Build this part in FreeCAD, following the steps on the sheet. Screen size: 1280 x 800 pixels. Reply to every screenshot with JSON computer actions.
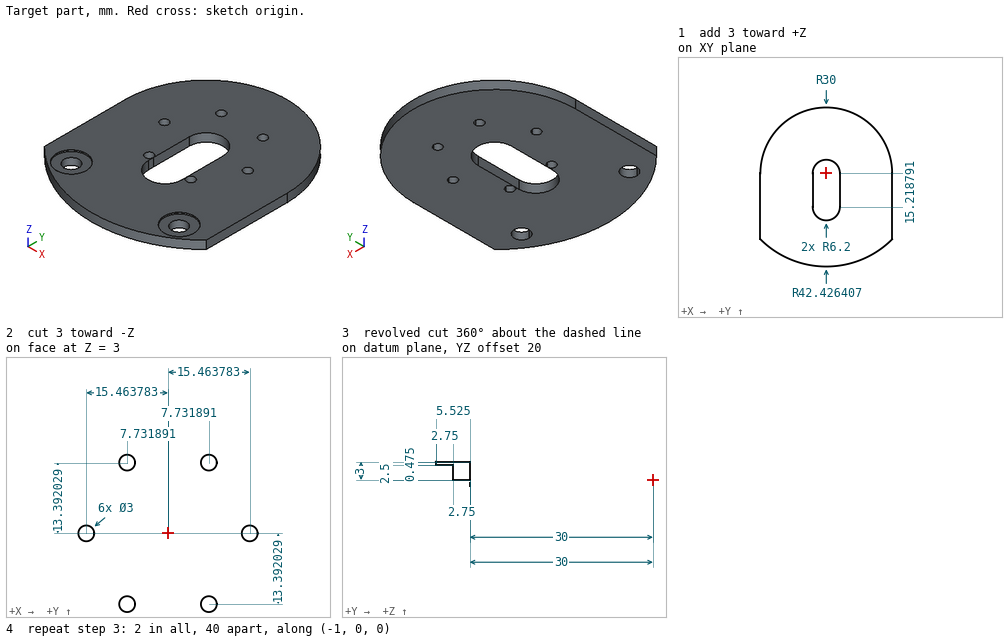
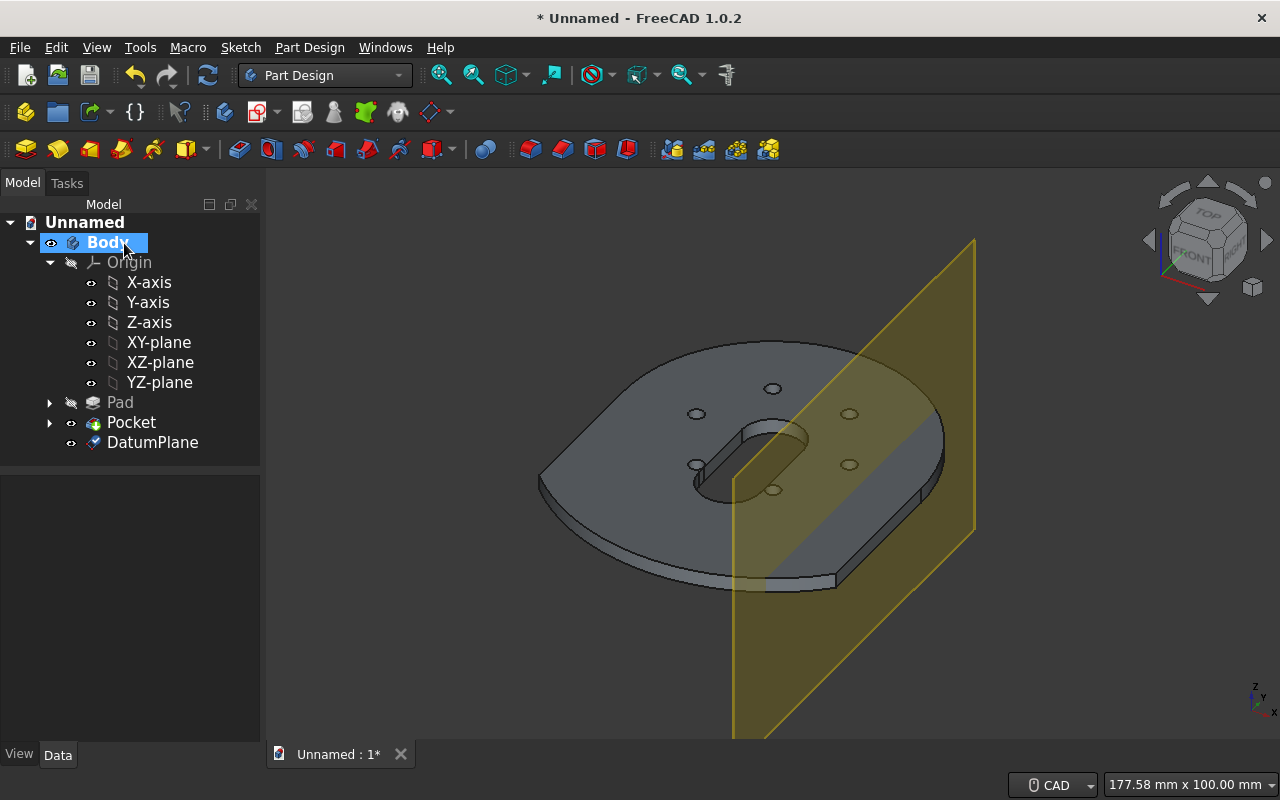
{"action": "left_click", "coordinate": [116, 443]}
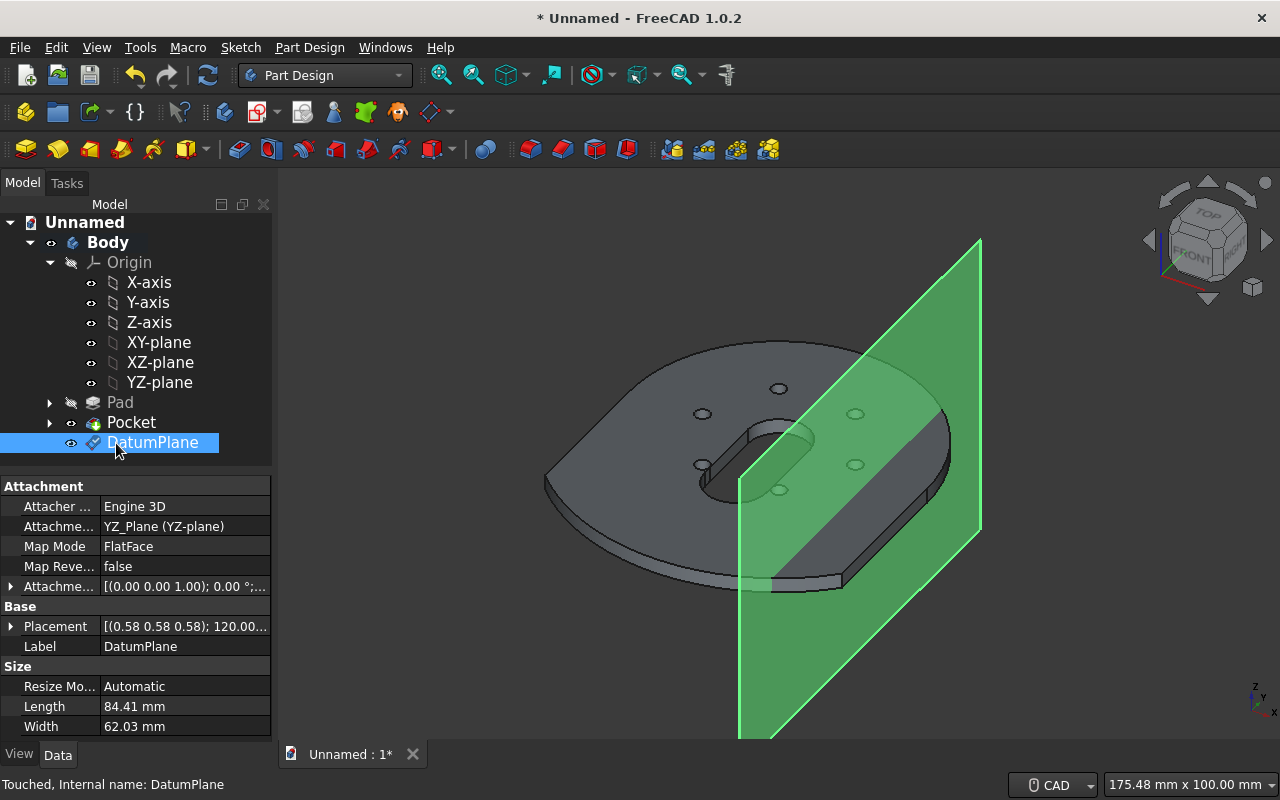
{"action": "left_click", "coordinate": [258, 112]}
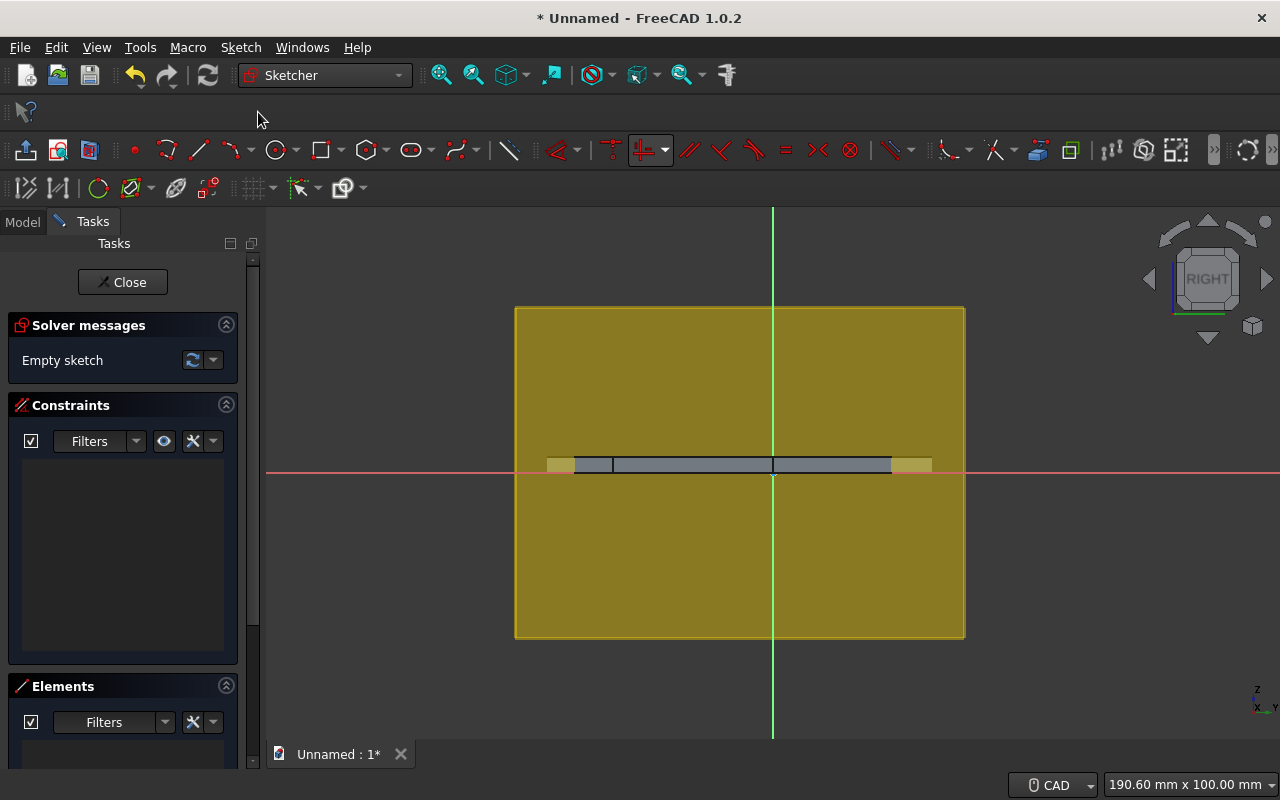
{"action": "left_click", "coordinate": [90, 150]}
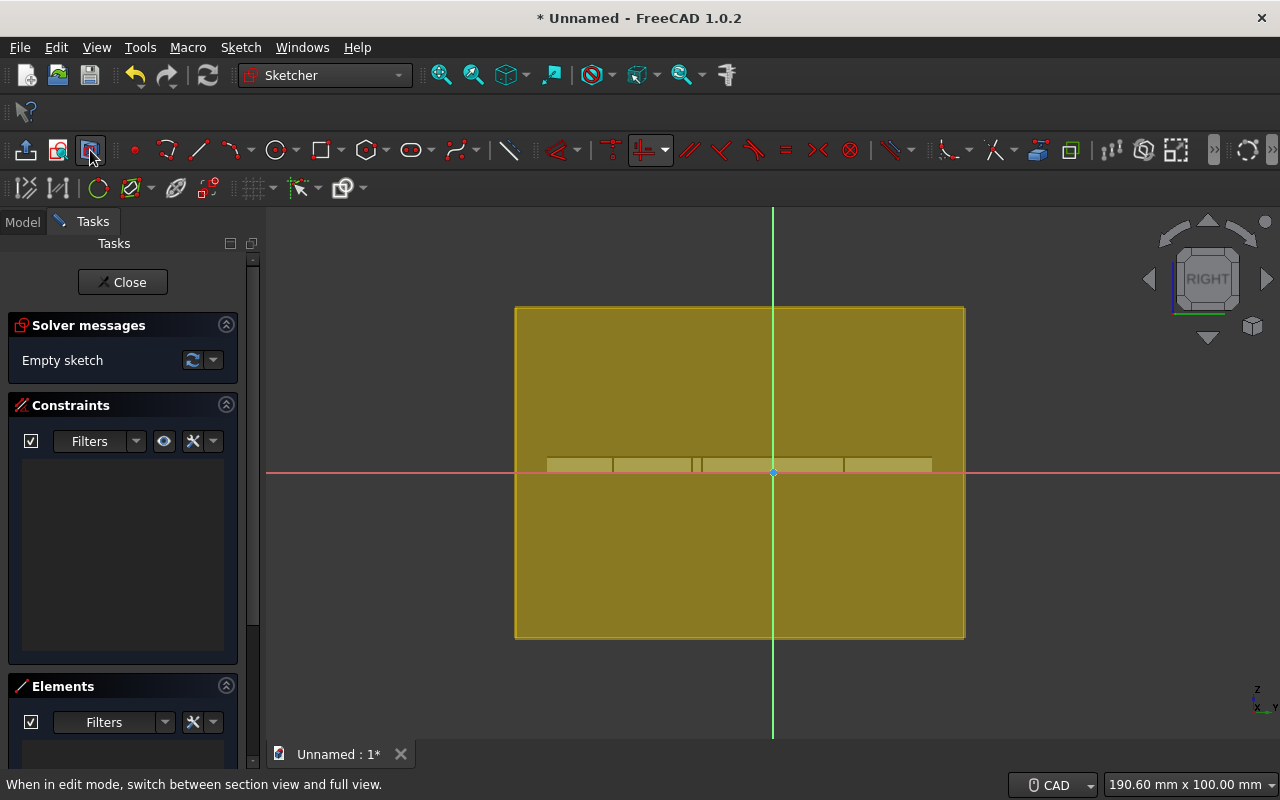
{"action": "scroll", "coordinate": [592, 468], "scroll_direction": "up", "scroll_amount": 14}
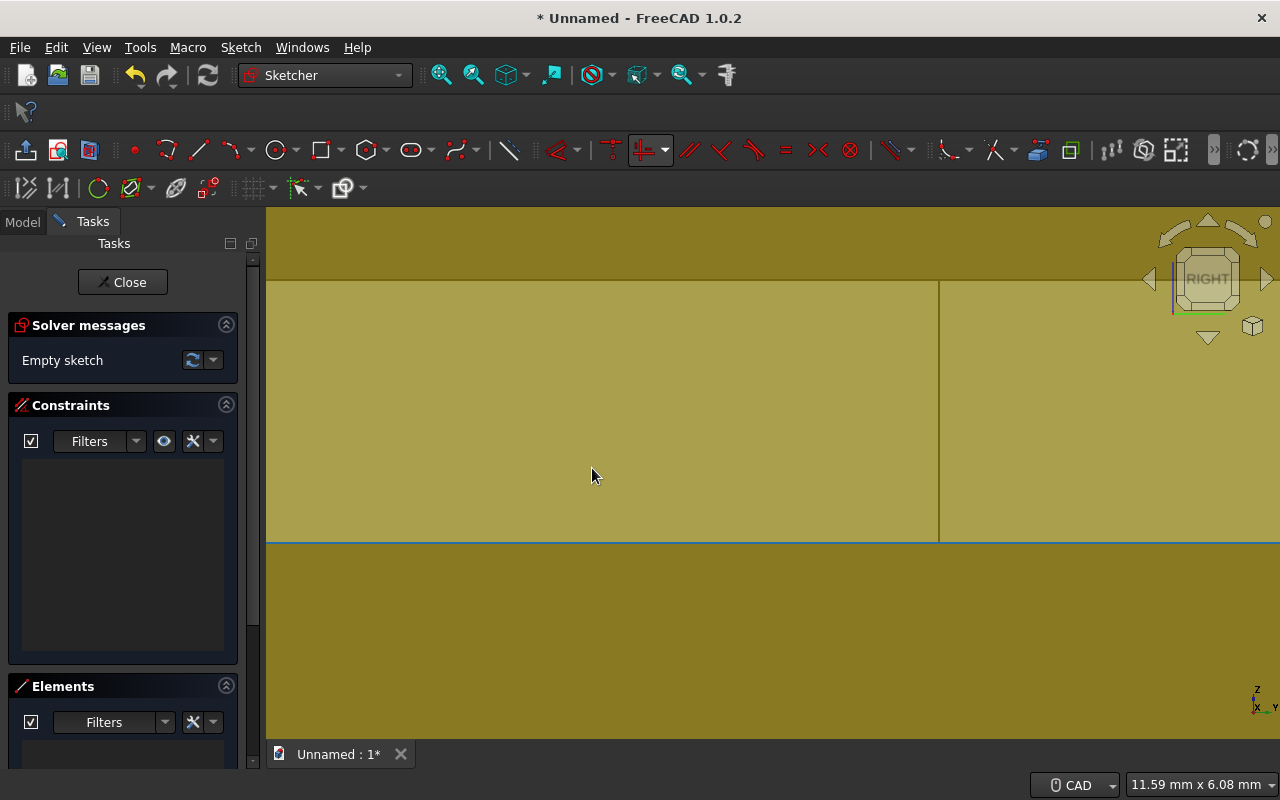
{"action": "key", "text": "g m"}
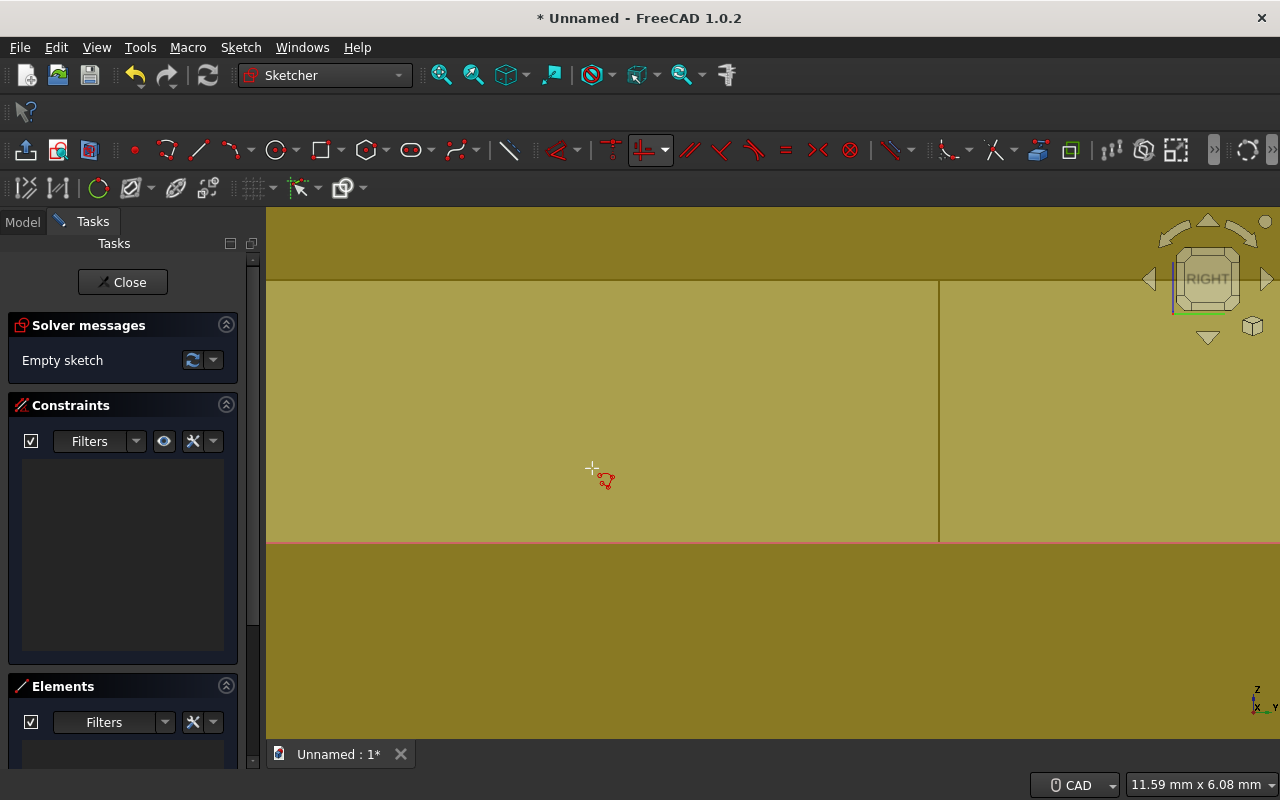
{"action": "left_click", "coordinate": [939, 543]}
{"action": "left_click", "coordinate": [939, 280]}
{"action": "left_click", "coordinate": [456, 280]}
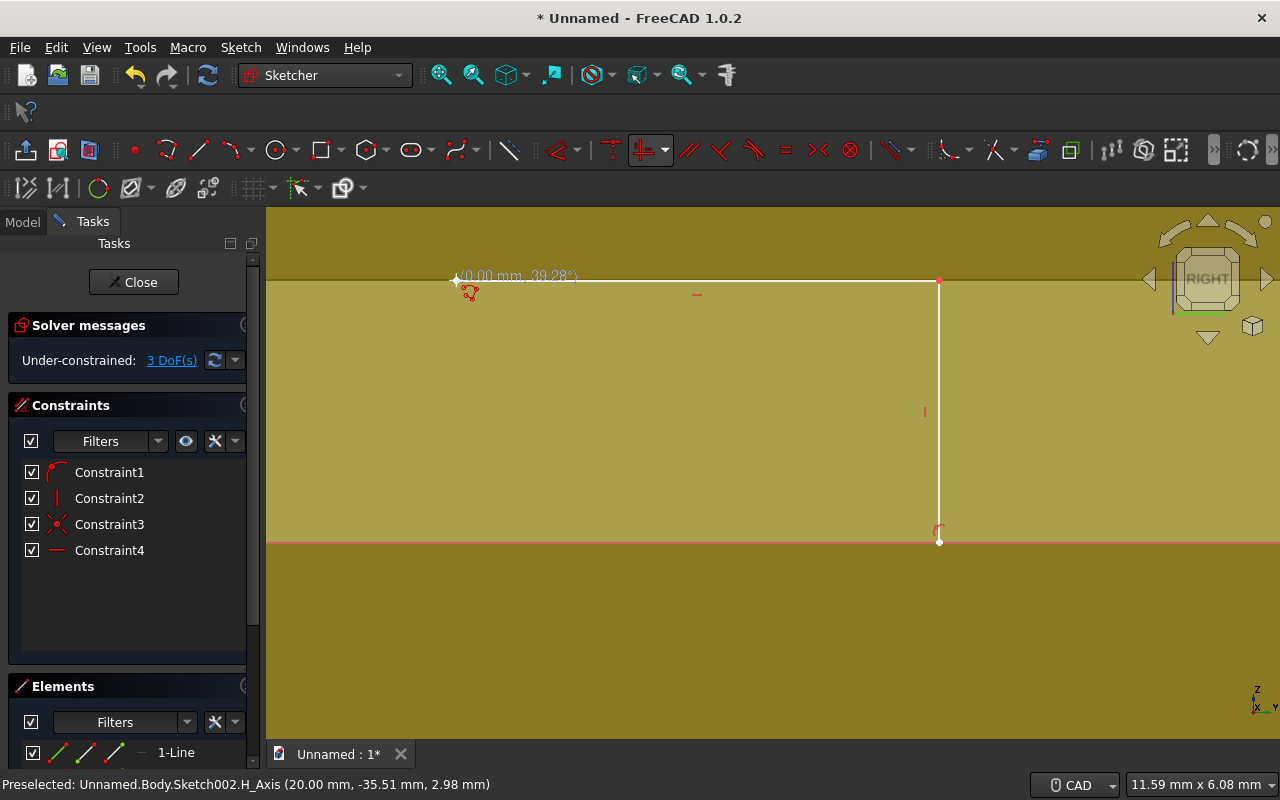
{"action": "scroll", "coordinate": [458, 282], "scroll_direction": "up", "scroll_amount": 10}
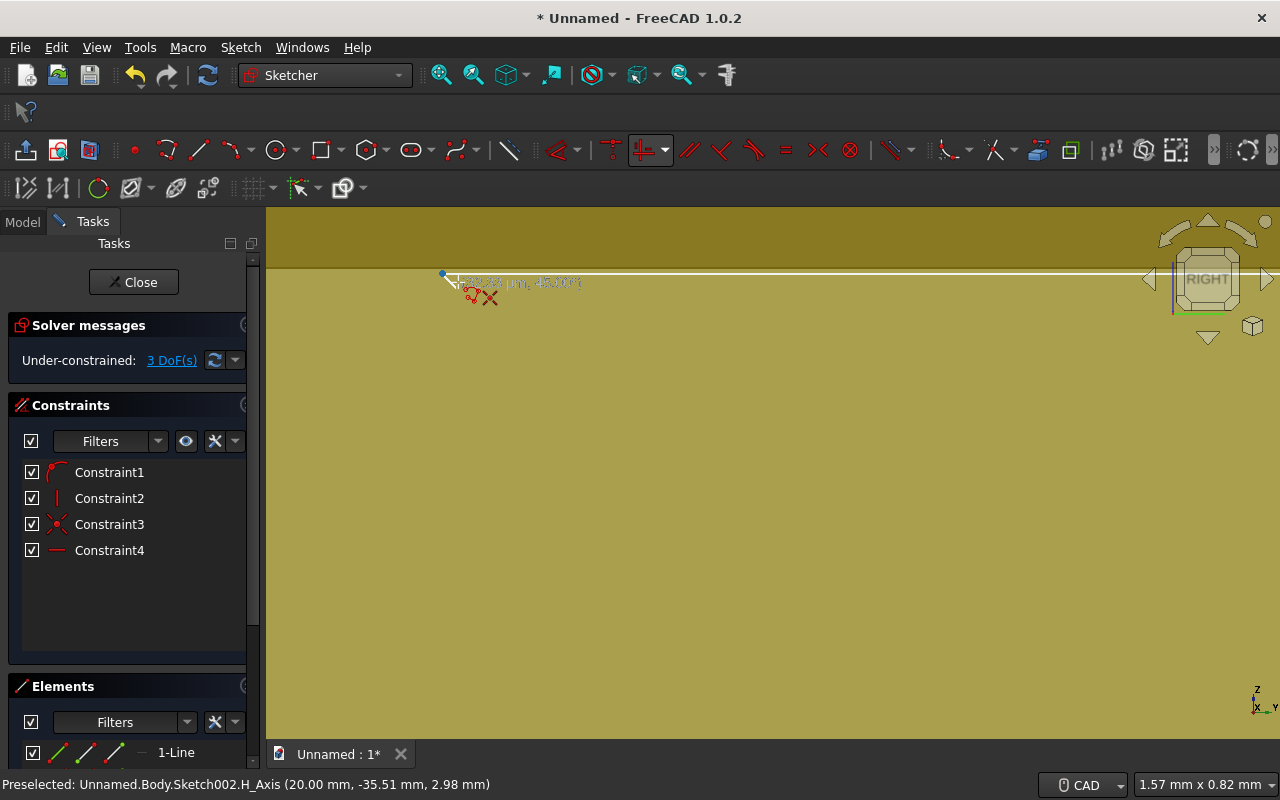
{"action": "left_click", "coordinate": [455, 284]}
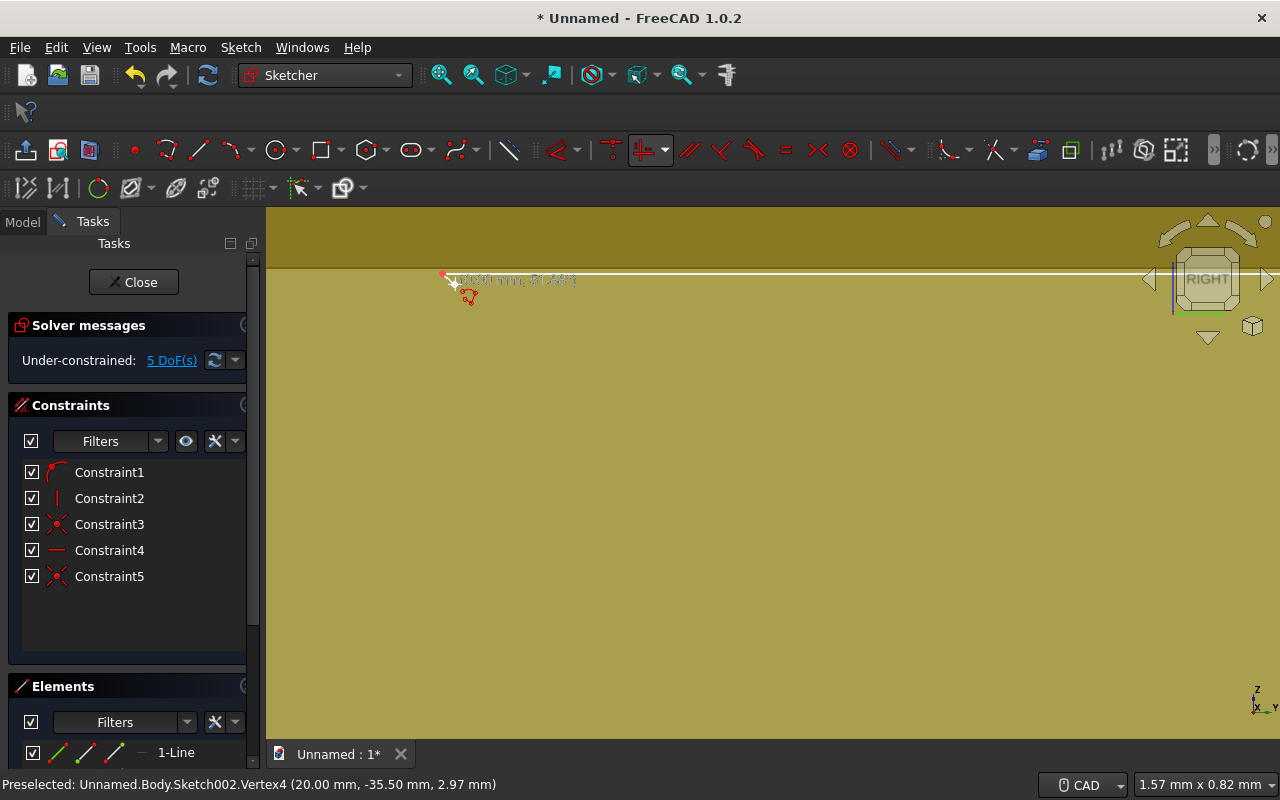
{"action": "scroll", "coordinate": [467, 293], "scroll_direction": "down", "scroll_amount": 10}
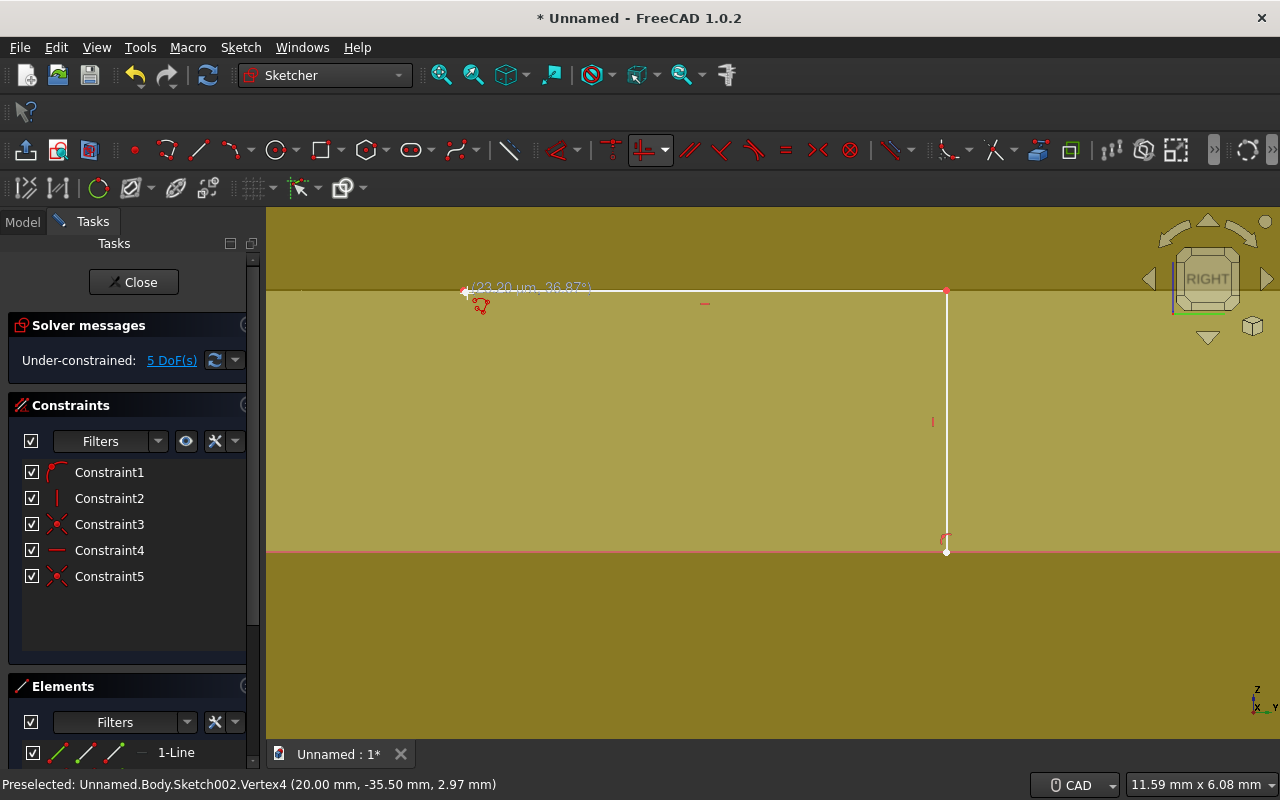
{"action": "left_click", "coordinate": [466, 333]}
{"action": "left_click", "coordinate": [706, 333]}
{"action": "left_click", "coordinate": [706, 543]}
{"action": "left_click", "coordinate": [947, 552]}